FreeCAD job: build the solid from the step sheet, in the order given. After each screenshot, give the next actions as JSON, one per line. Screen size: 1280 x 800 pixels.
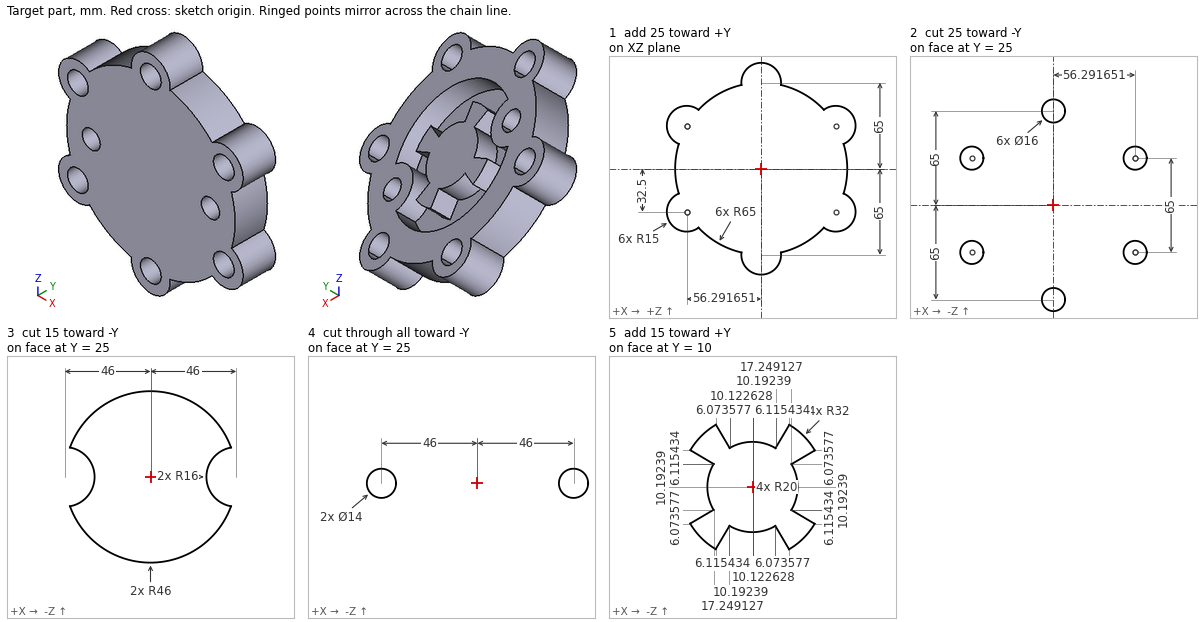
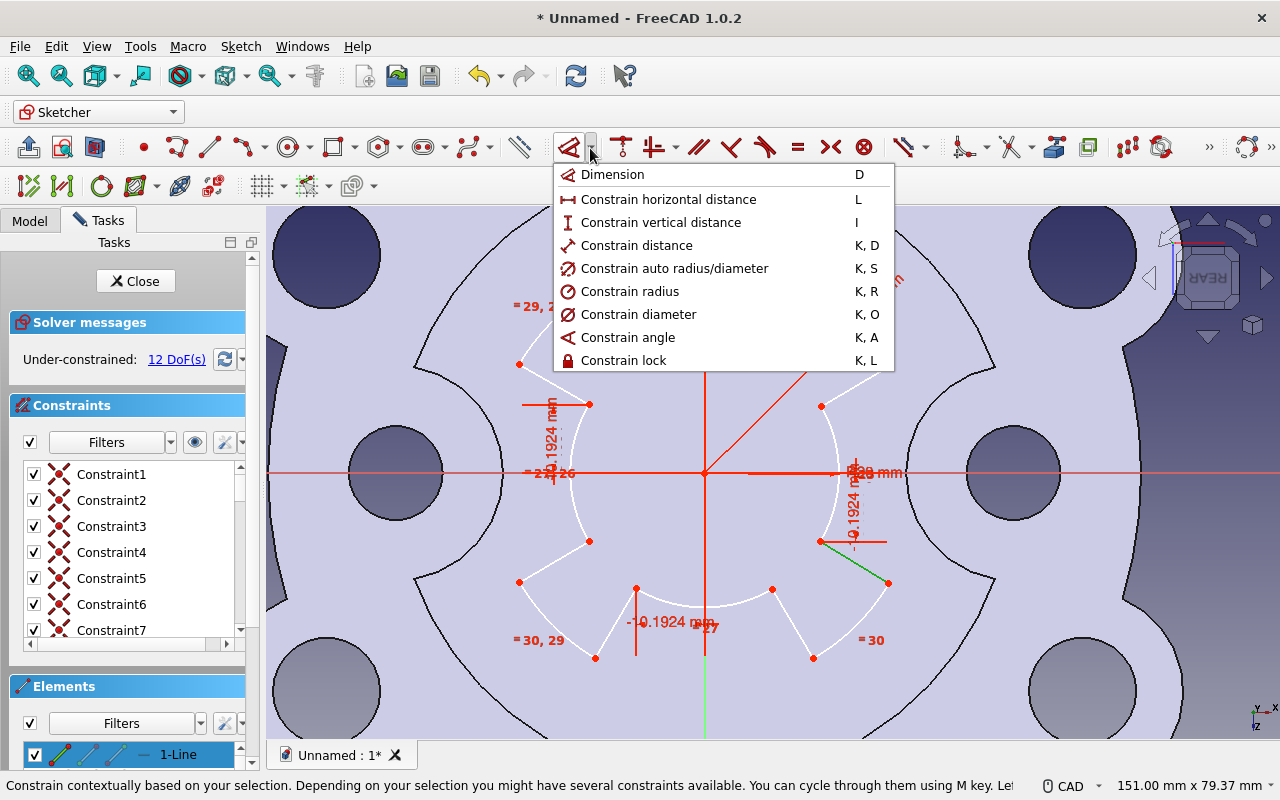
{"action": "left_click", "coordinate": [724, 222]}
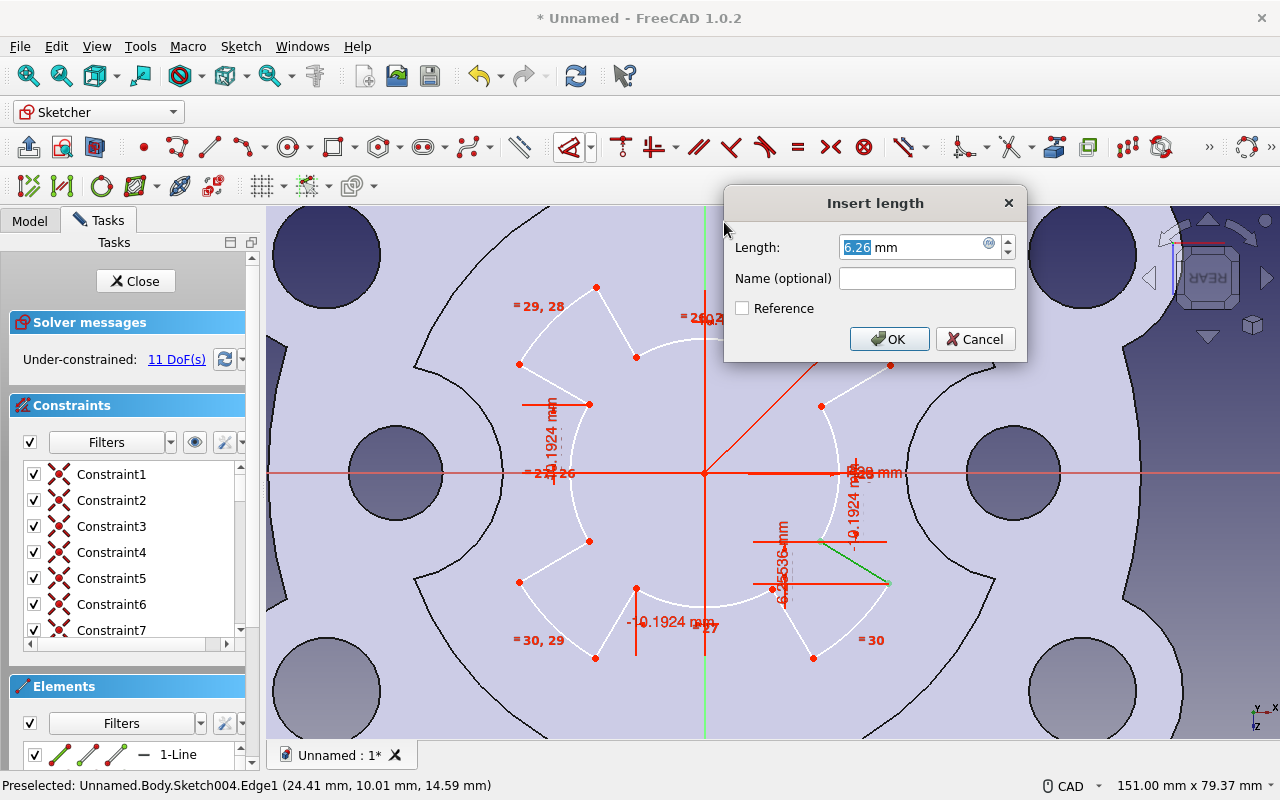
{"action": "type", "text": "6.115434"}
{"action": "key", "text": "Return"}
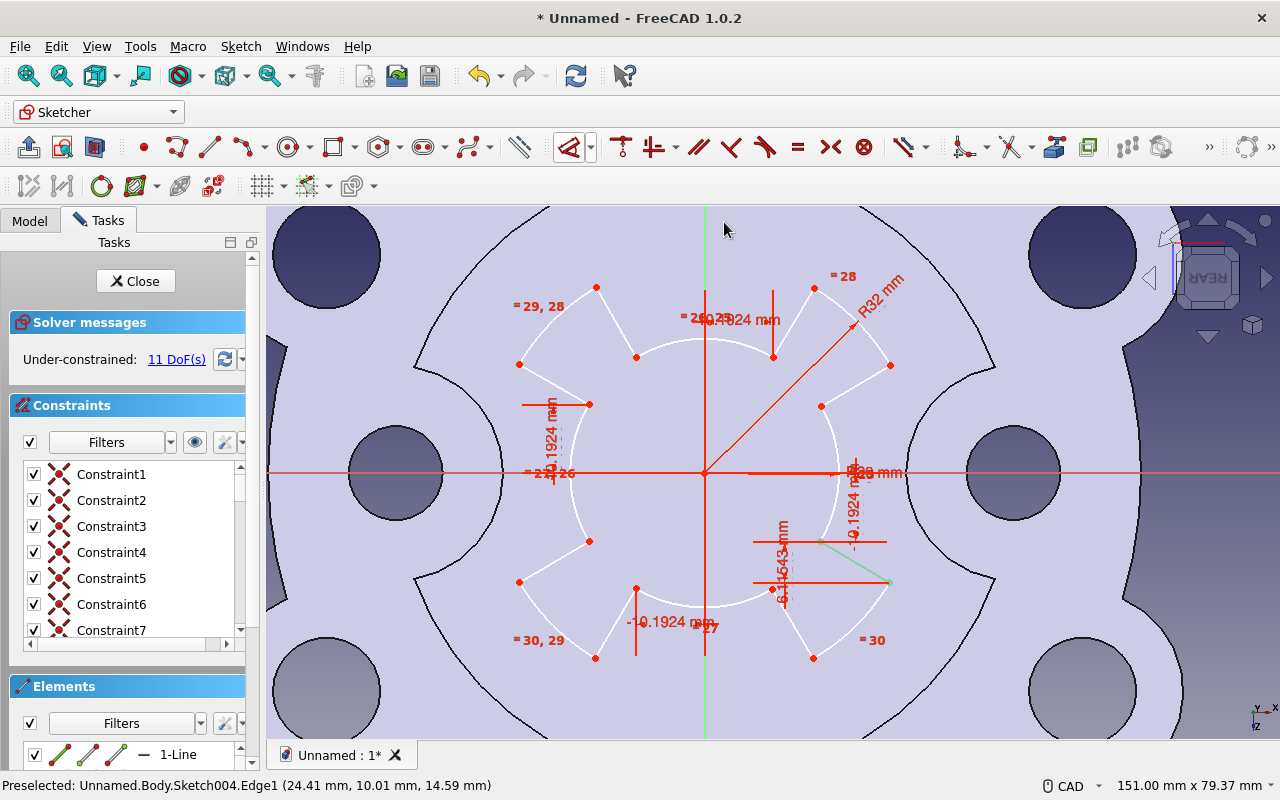
{"action": "left_click", "coordinate": [842, 394]}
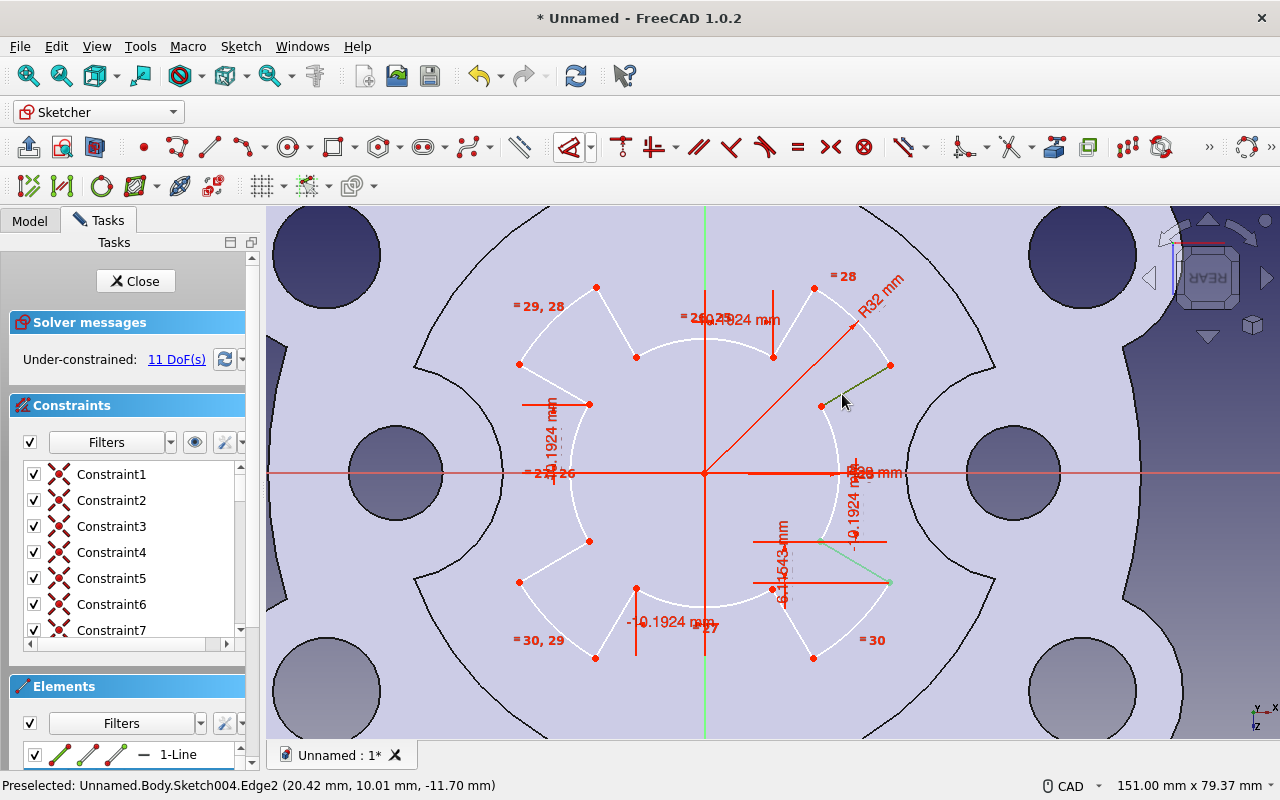
{"action": "left_click", "coordinate": [590, 148]}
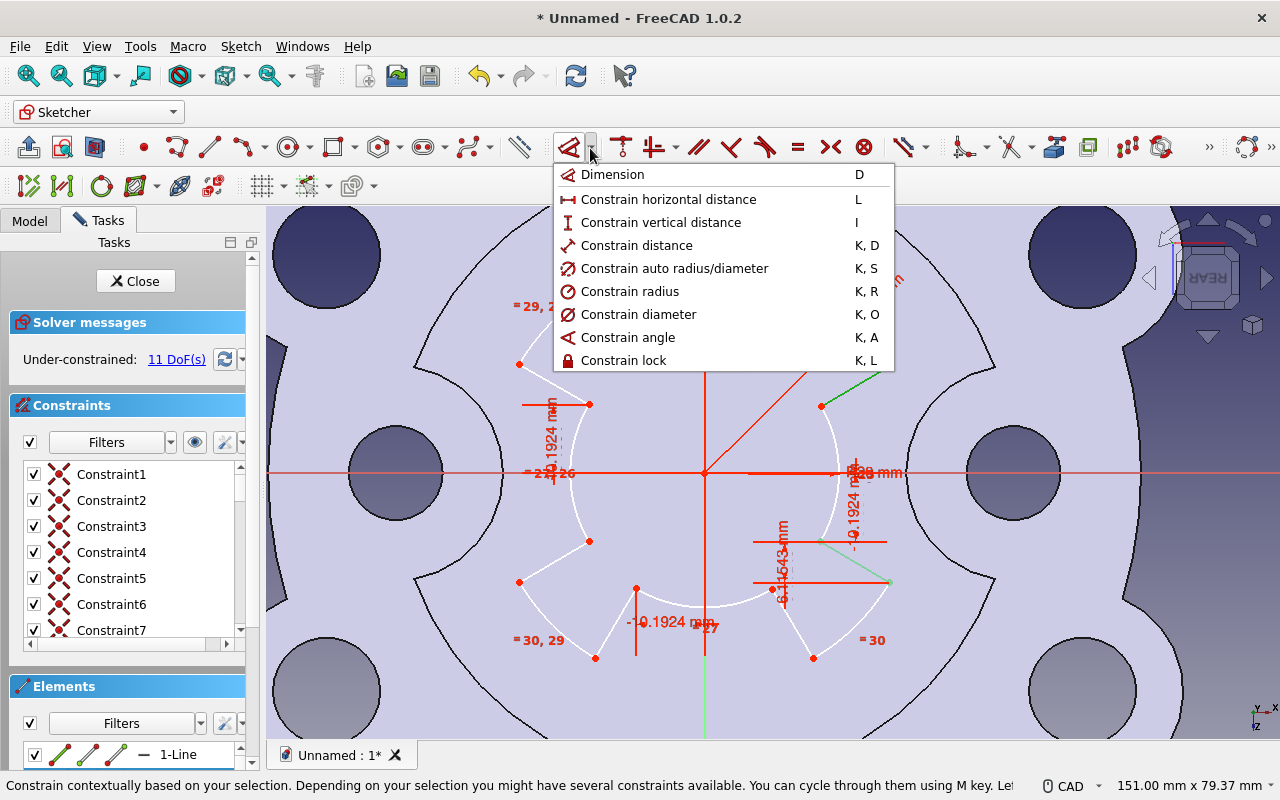
{"action": "left_click", "coordinate": [724, 222]}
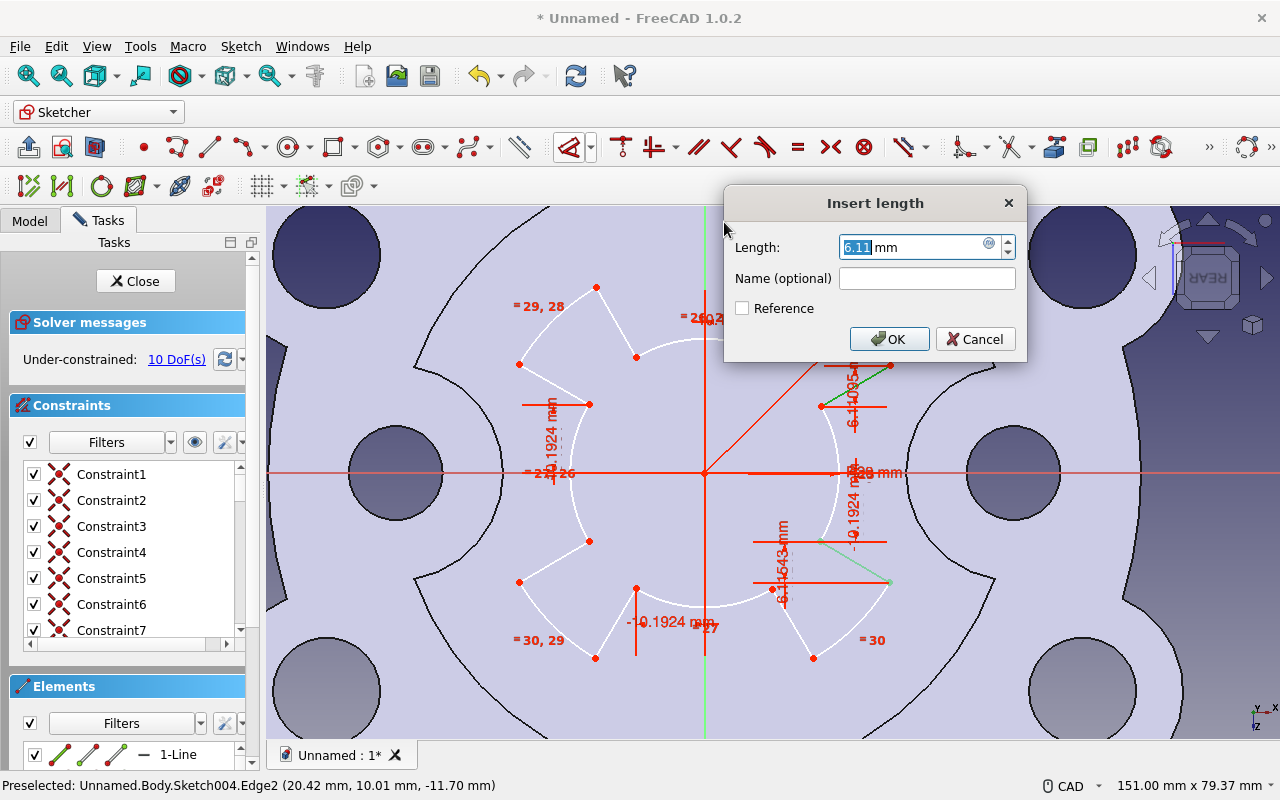
{"action": "type", "text": "6.073577"}
{"action": "key", "text": "Return"}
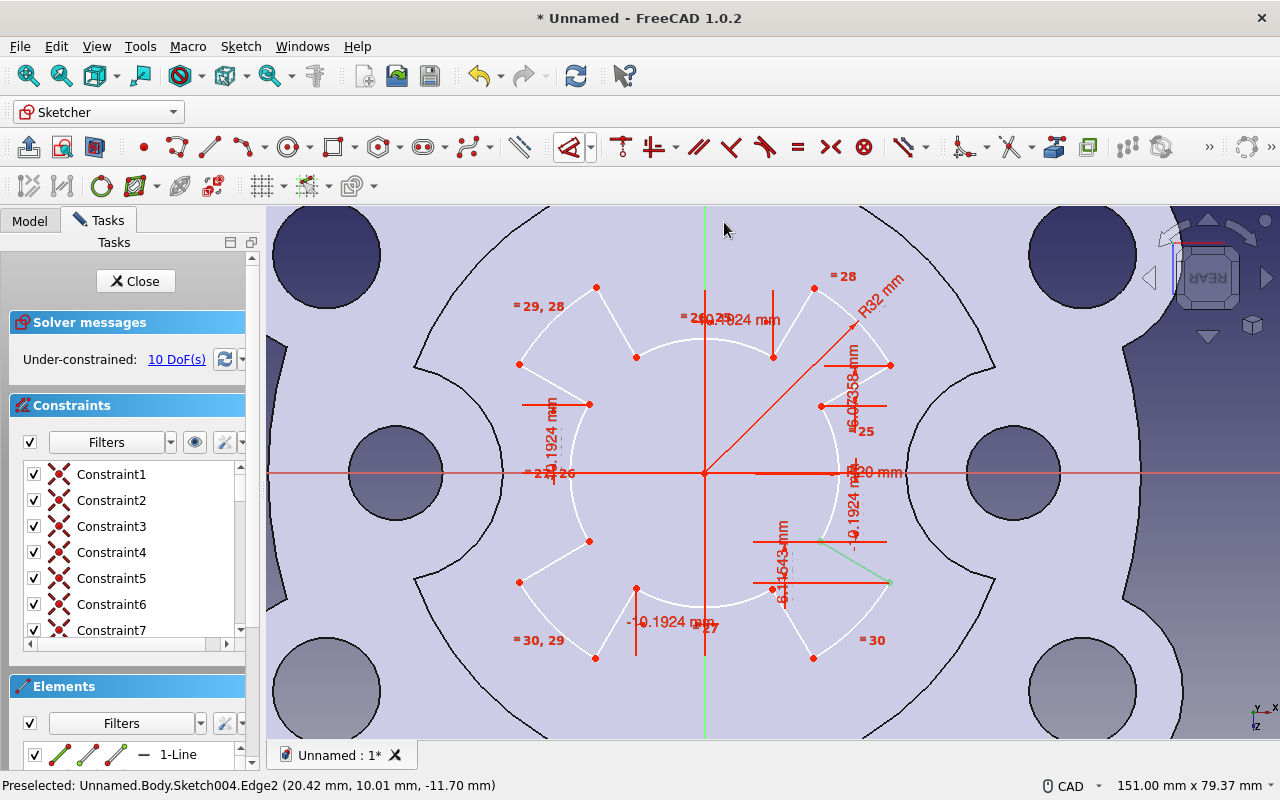
{"action": "left_click", "coordinate": [802, 309]}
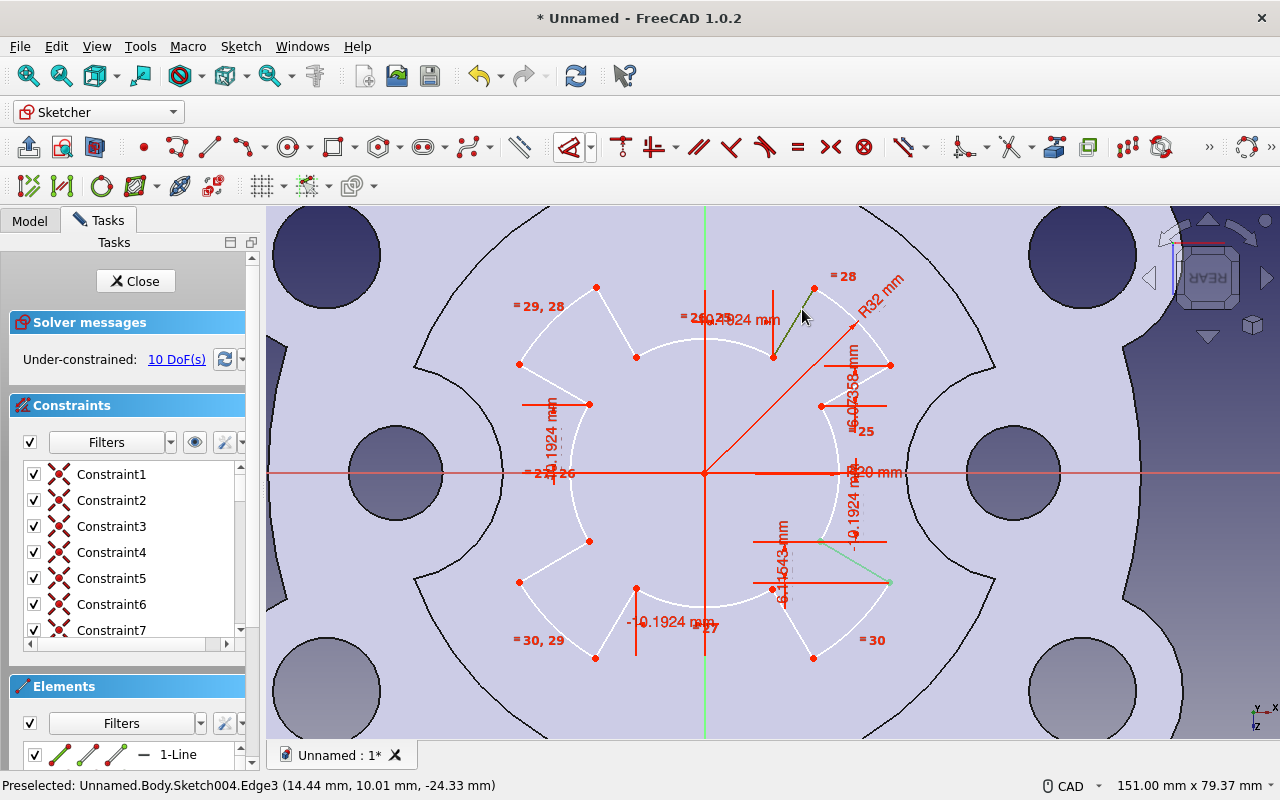
{"action": "left_click", "coordinate": [590, 148]}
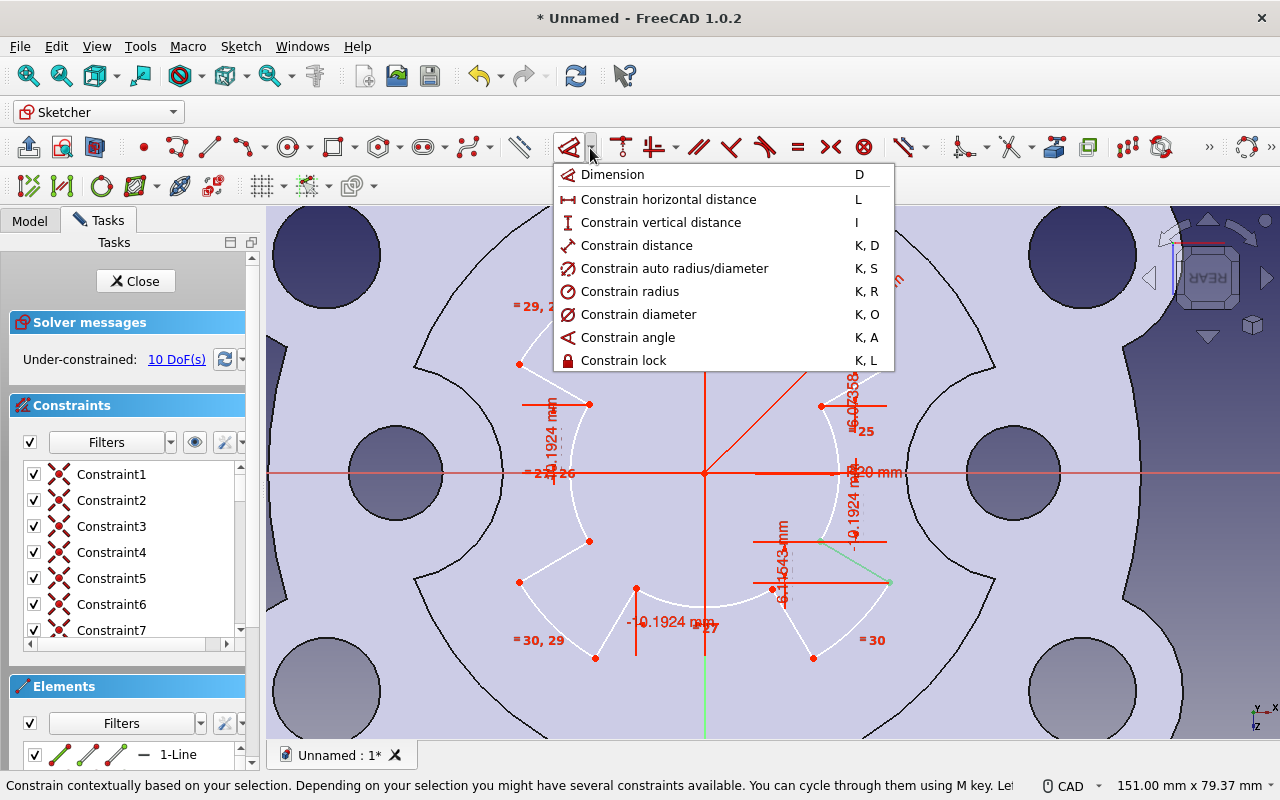
{"action": "left_click", "coordinate": [724, 200]}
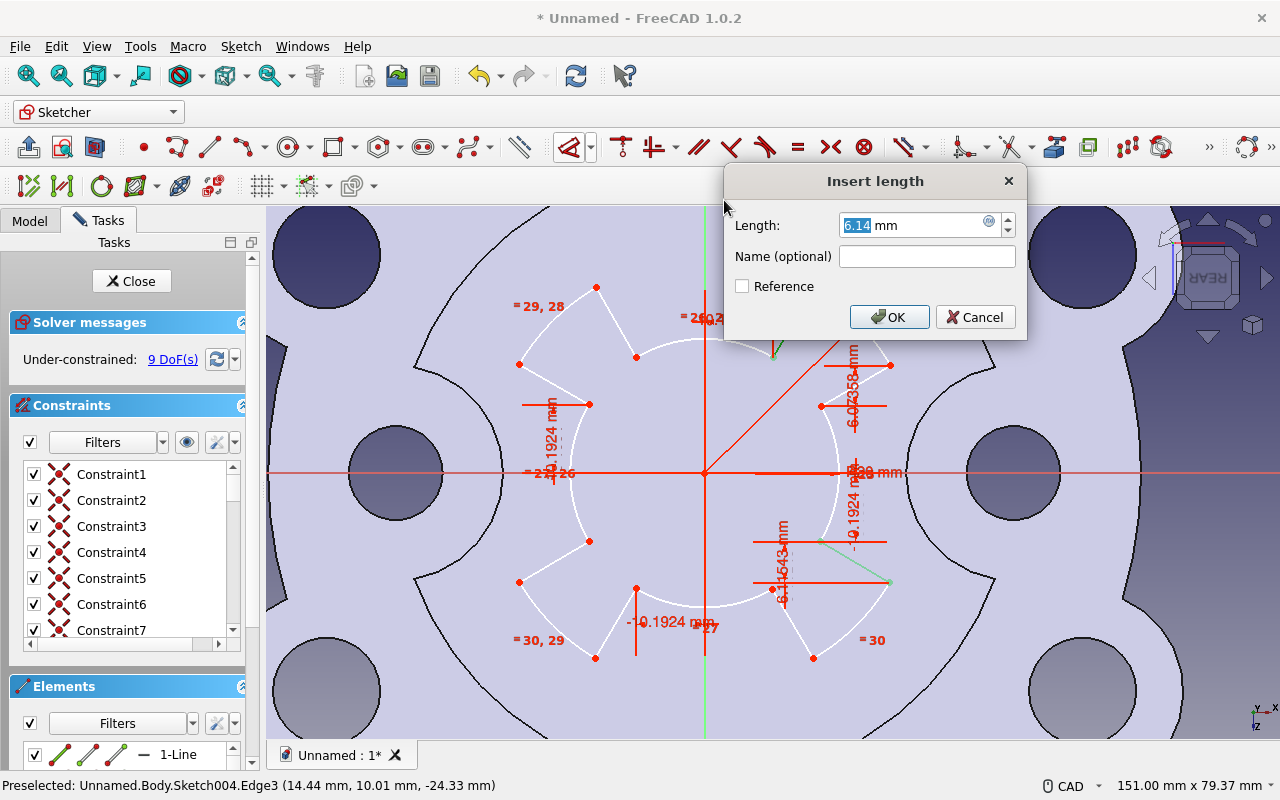
{"action": "type", "text": "6.115434"}
{"action": "key", "text": "Return"}